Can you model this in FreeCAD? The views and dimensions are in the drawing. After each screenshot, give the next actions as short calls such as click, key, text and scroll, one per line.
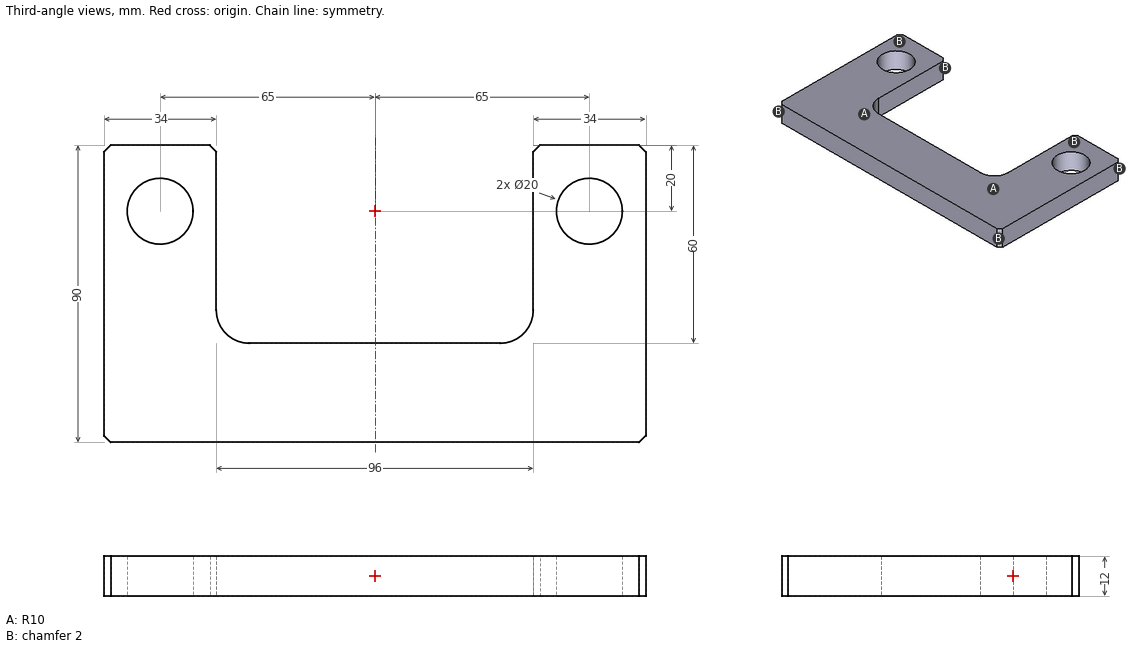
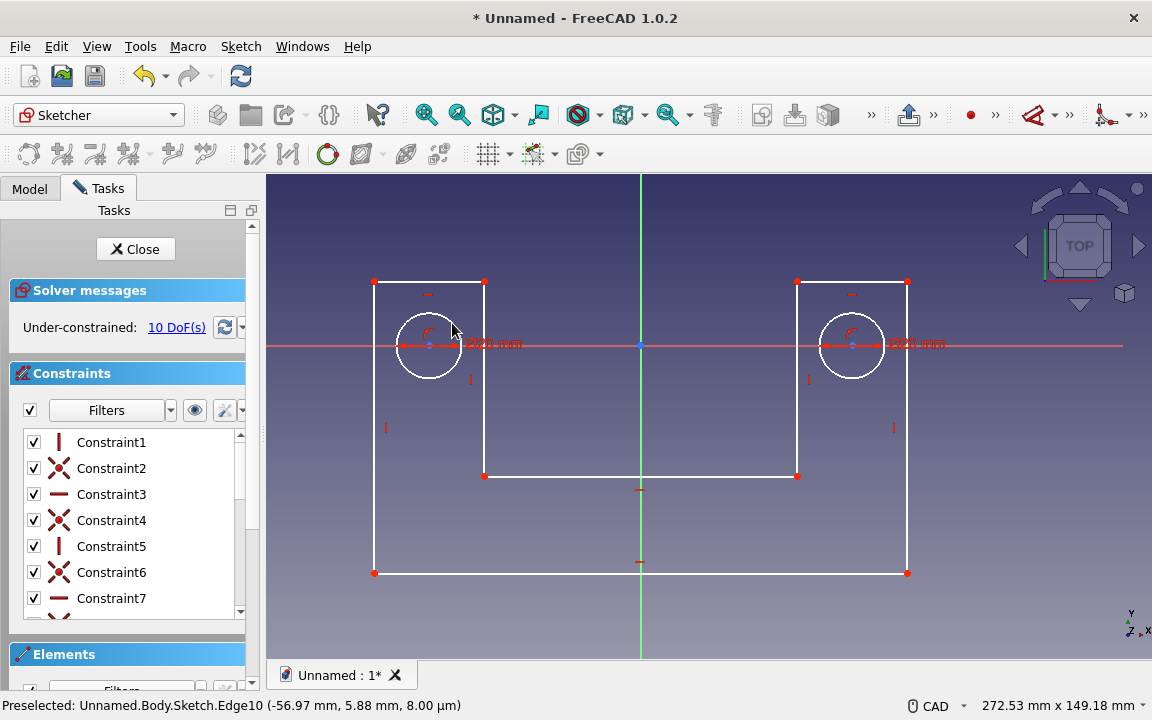
click(797, 282)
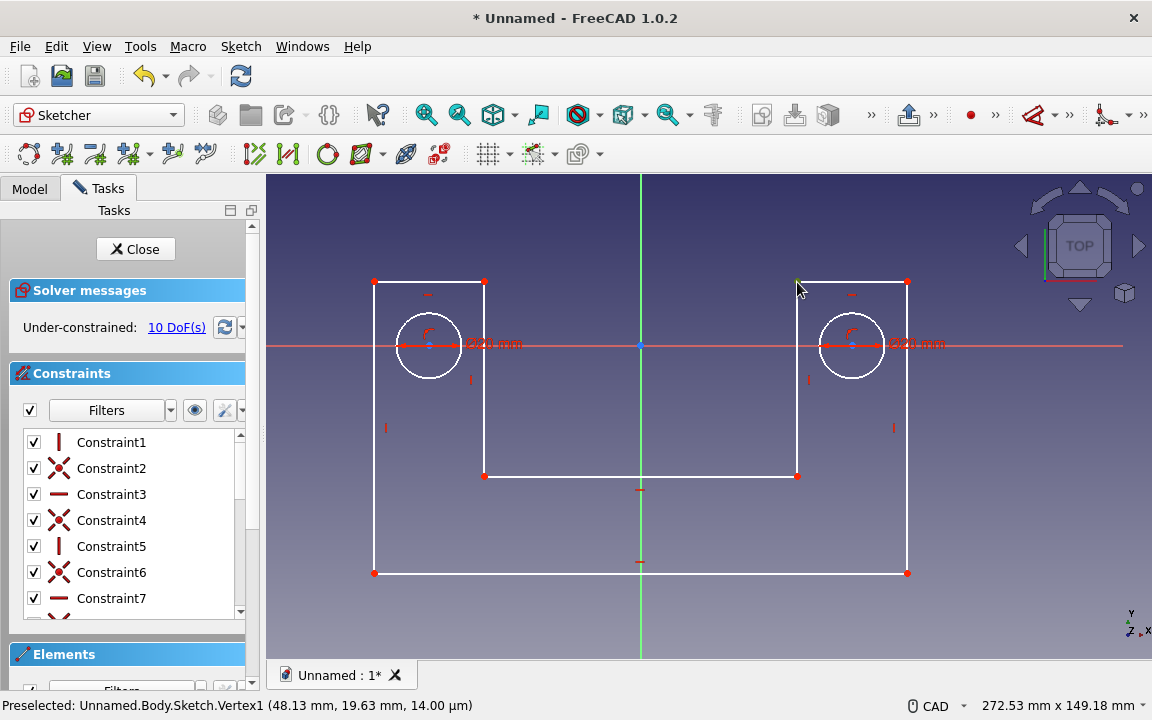
click(484, 282)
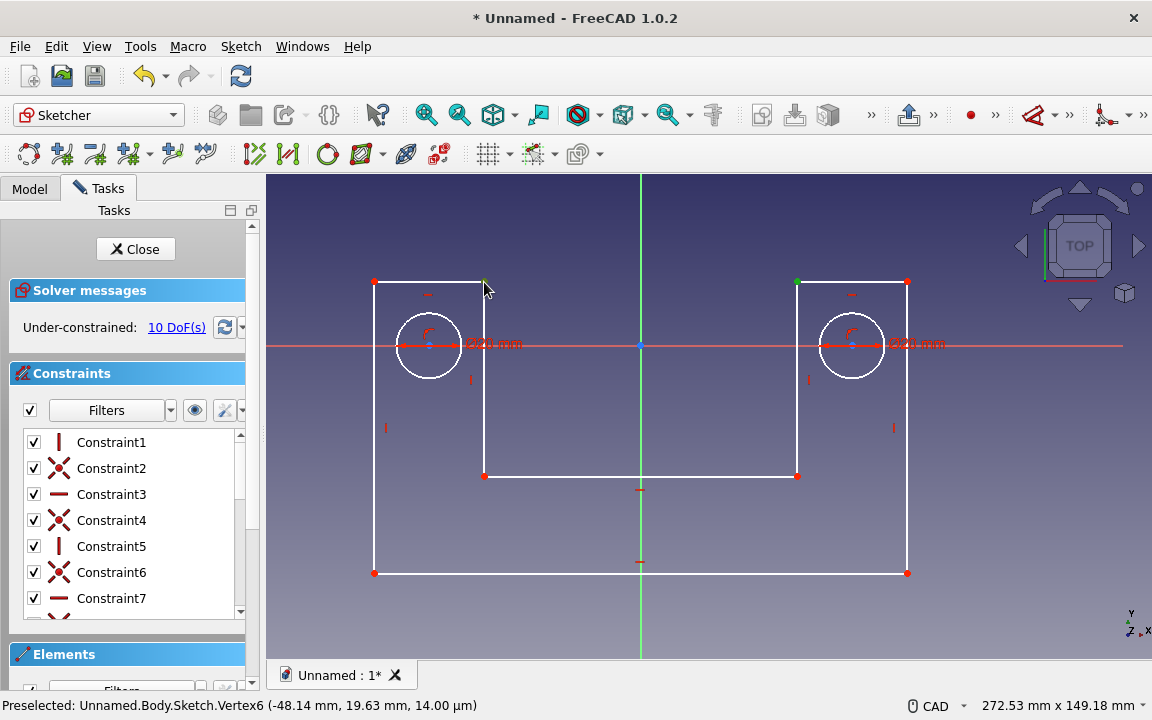
click(641, 539)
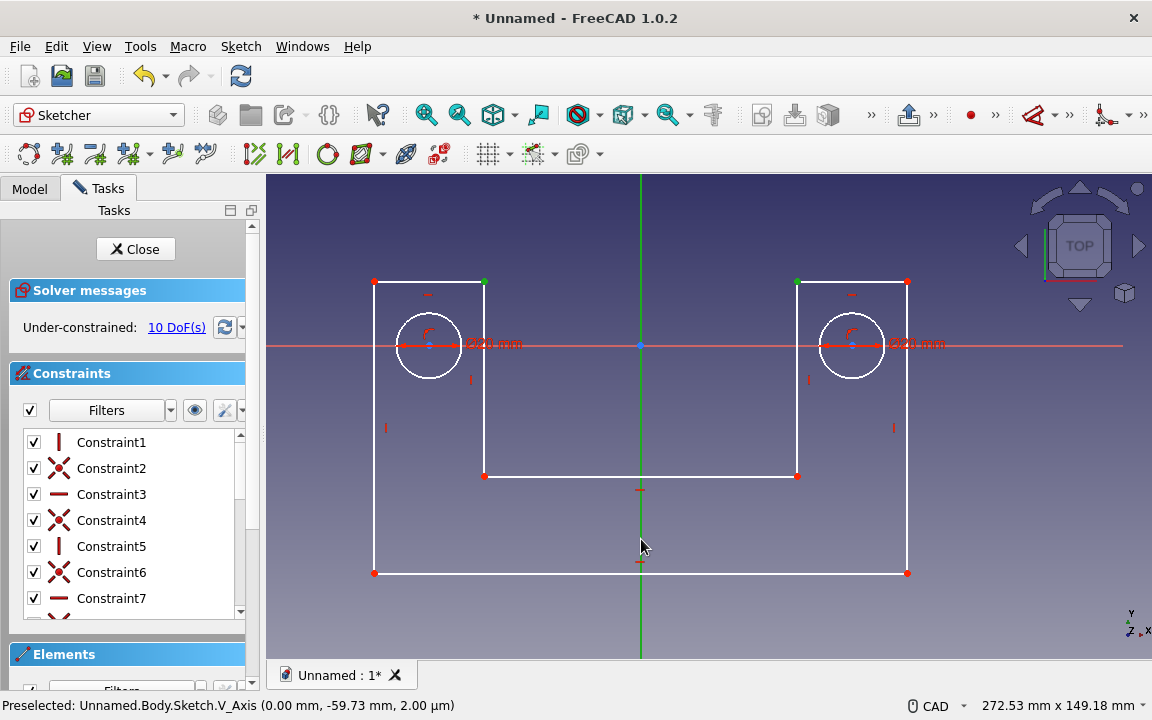
key(s)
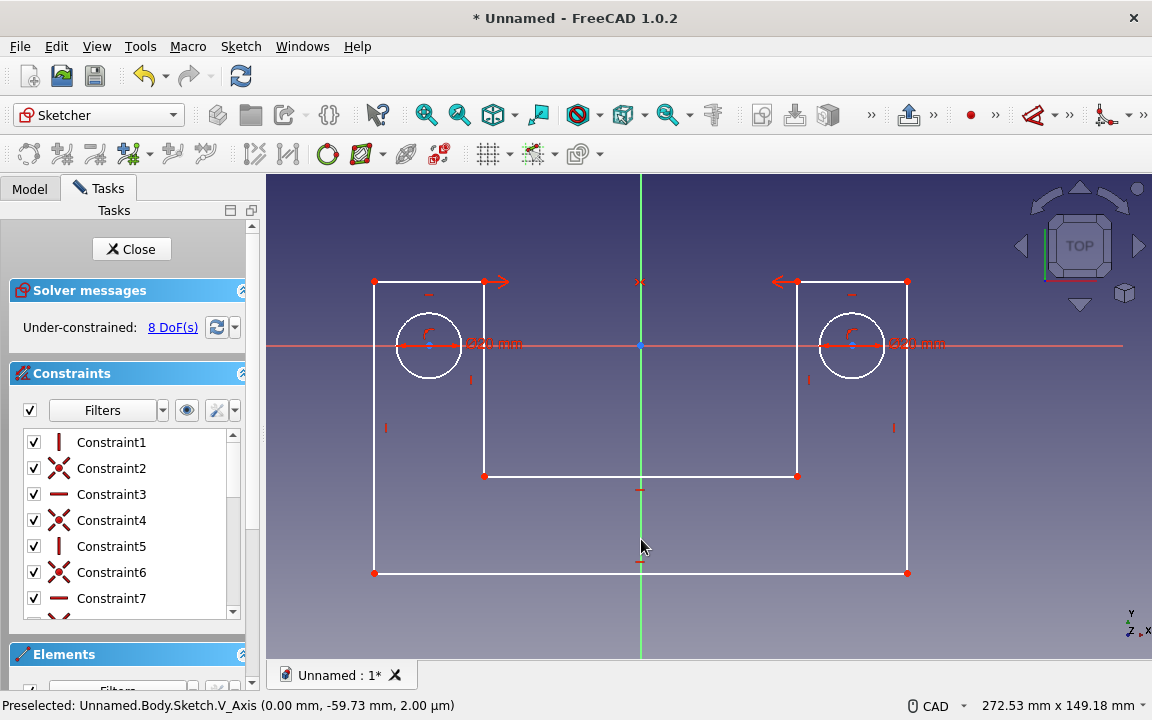
click(1032, 116)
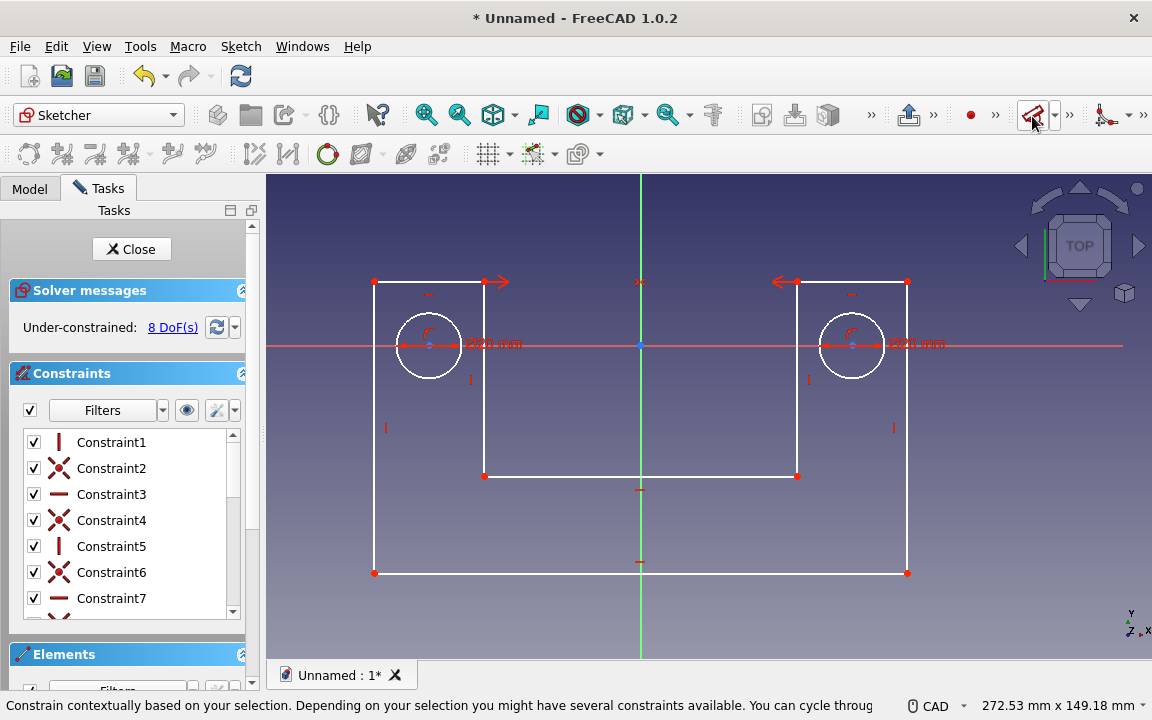
click(797, 418)
click(831, 424)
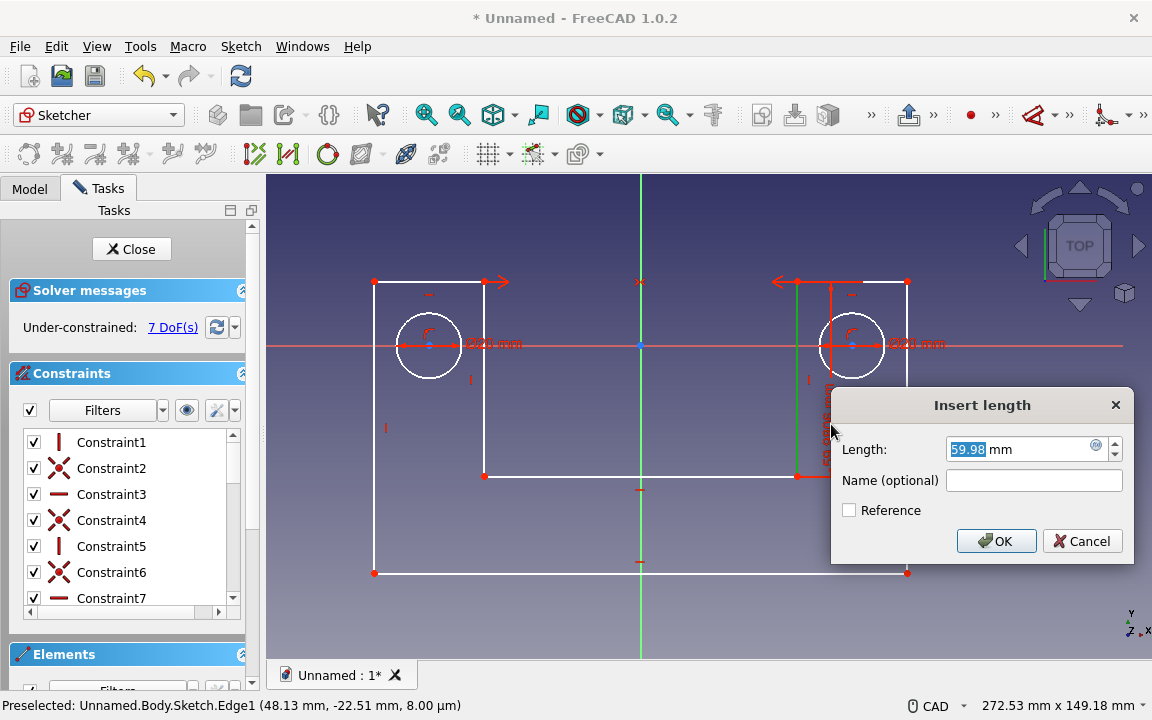
text(60)
key(Return)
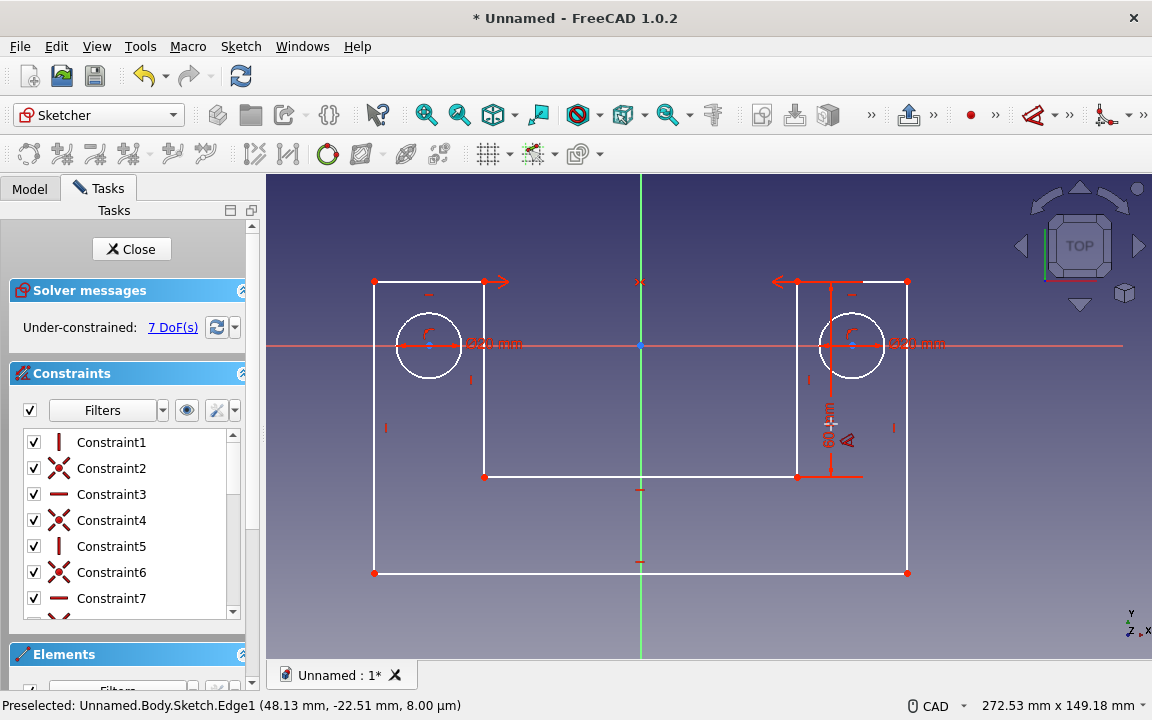
click(703, 477)
click(569, 511)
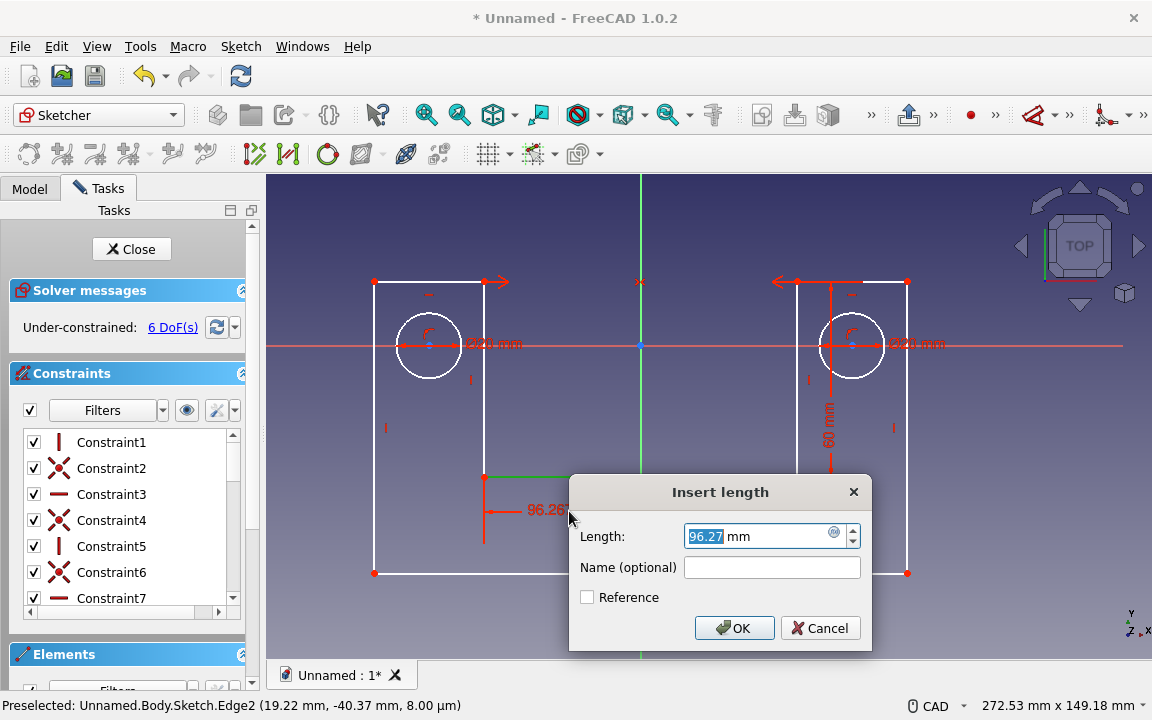
text(96)
key(Return)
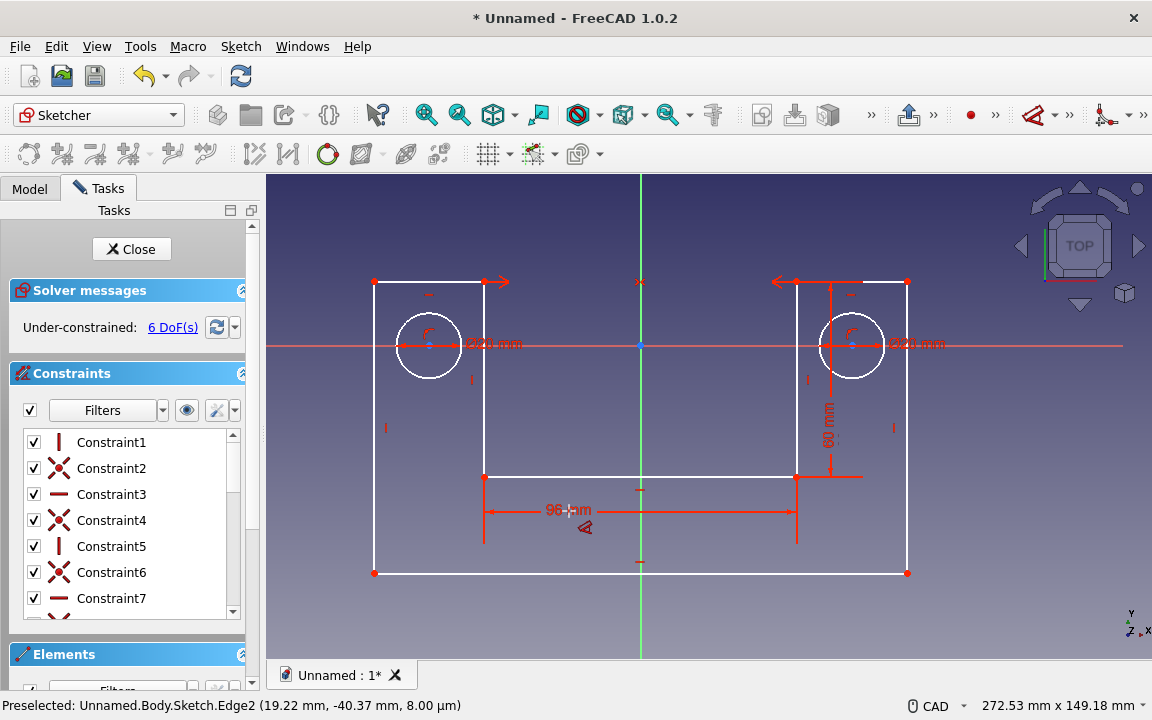
click(451, 282)
click(429, 248)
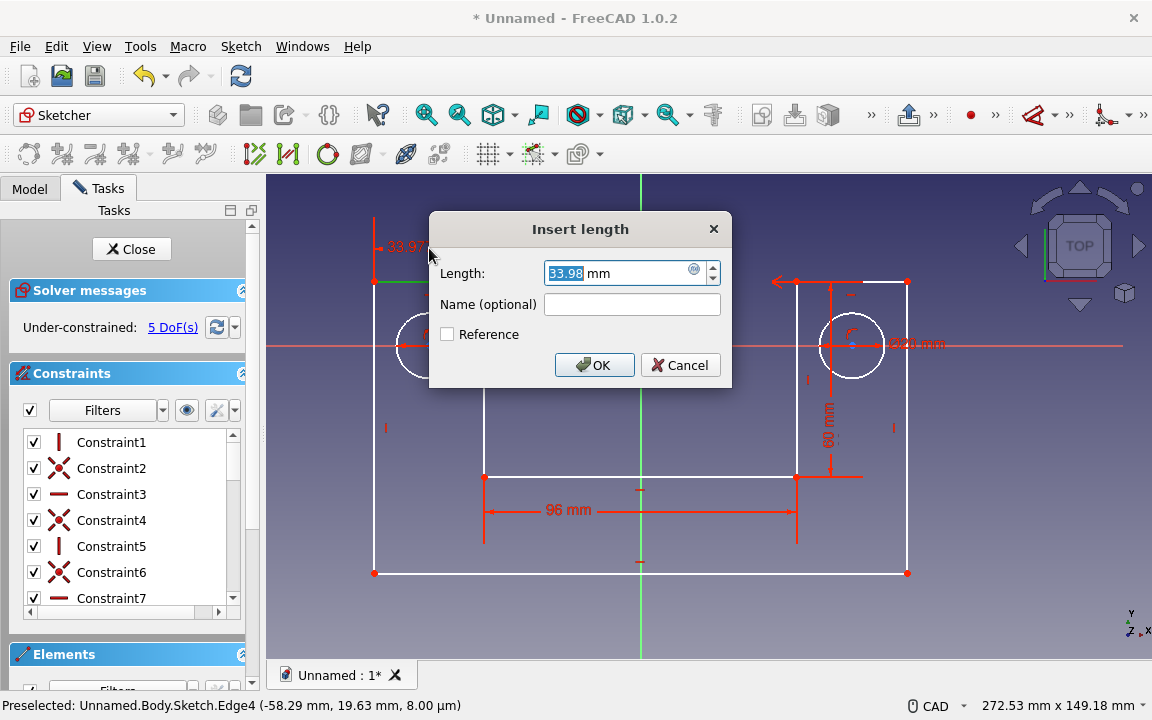
text(34)
key(Return)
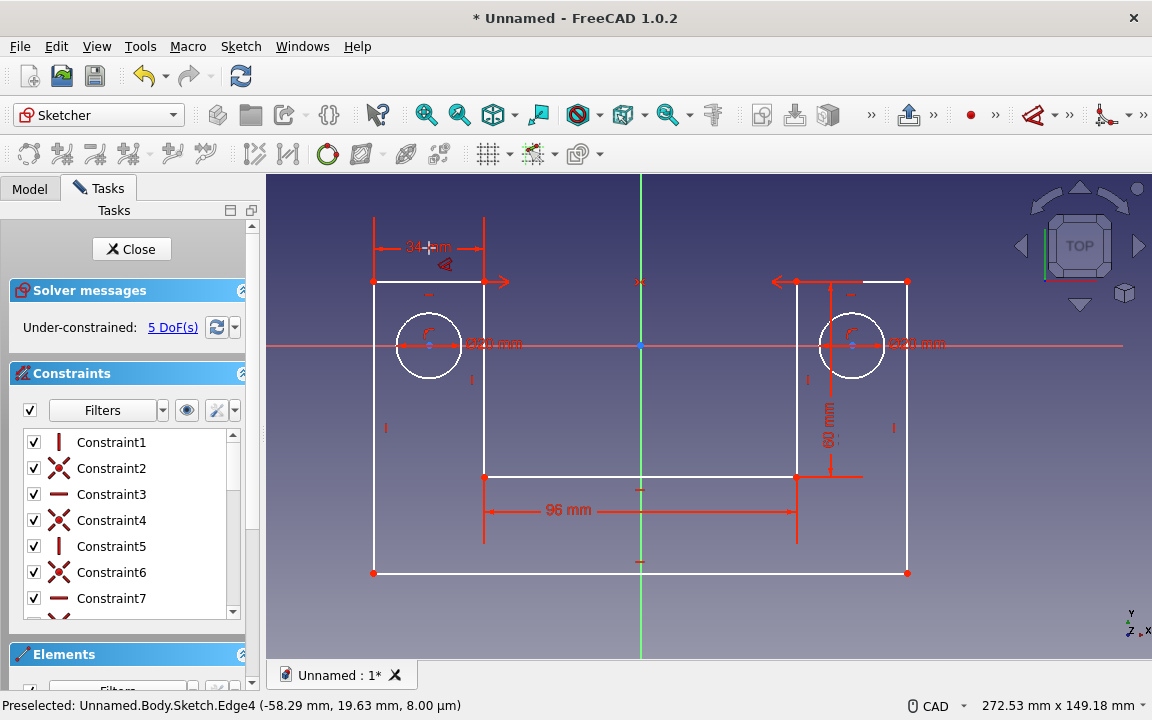
click(374, 370)
click(340, 428)